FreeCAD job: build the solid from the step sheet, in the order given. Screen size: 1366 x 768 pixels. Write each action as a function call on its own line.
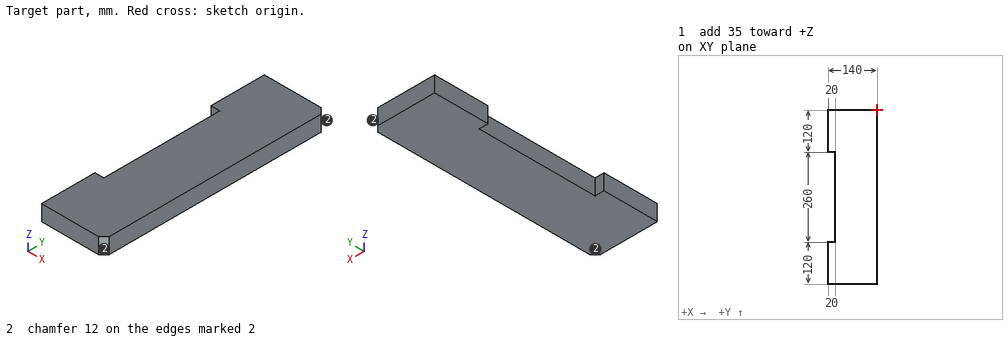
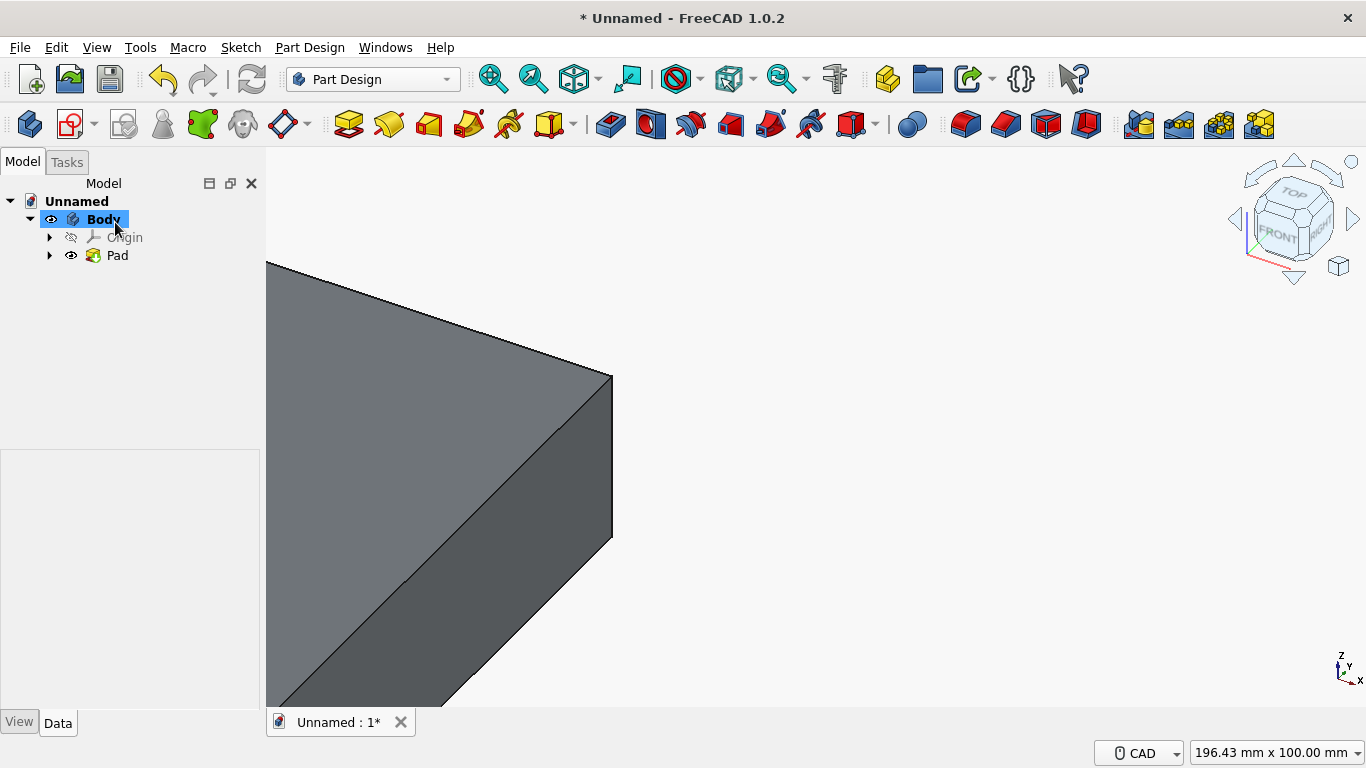
click(494, 80)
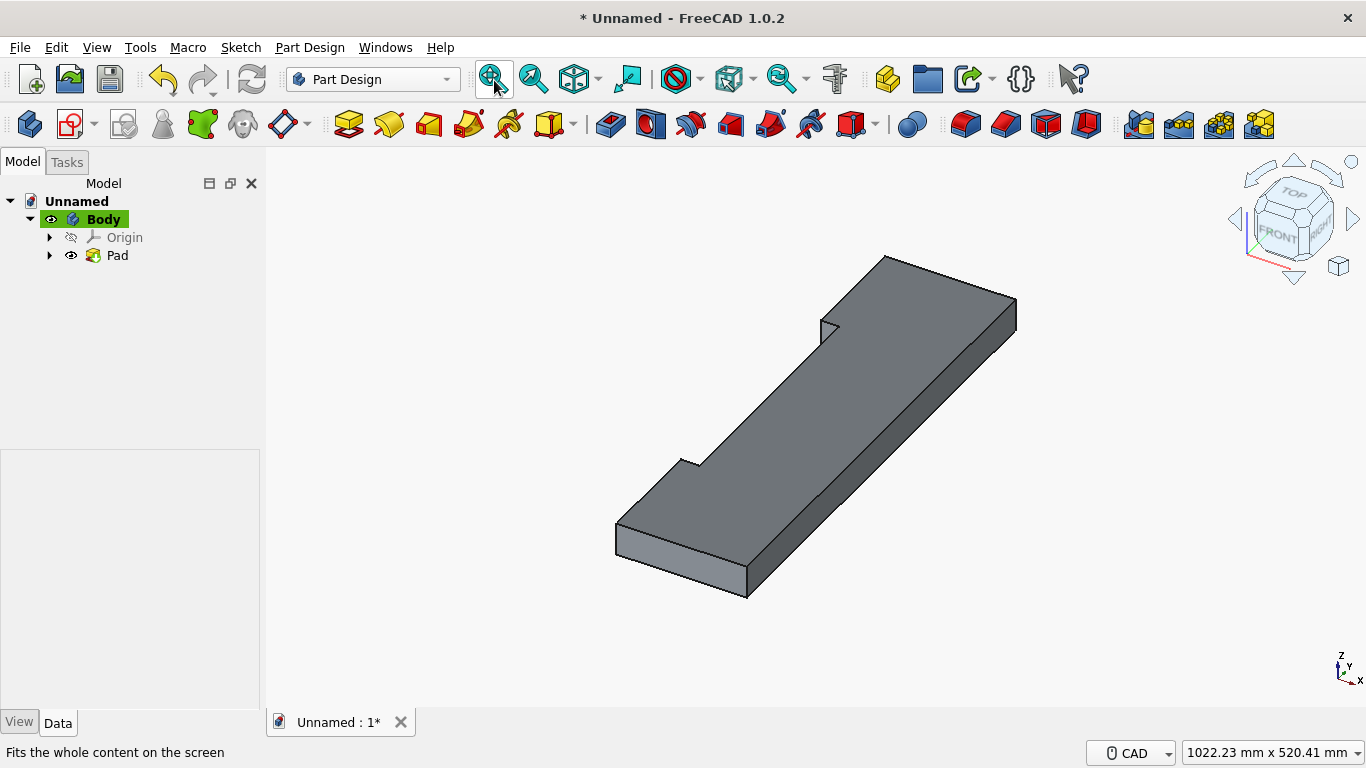
click(747, 581)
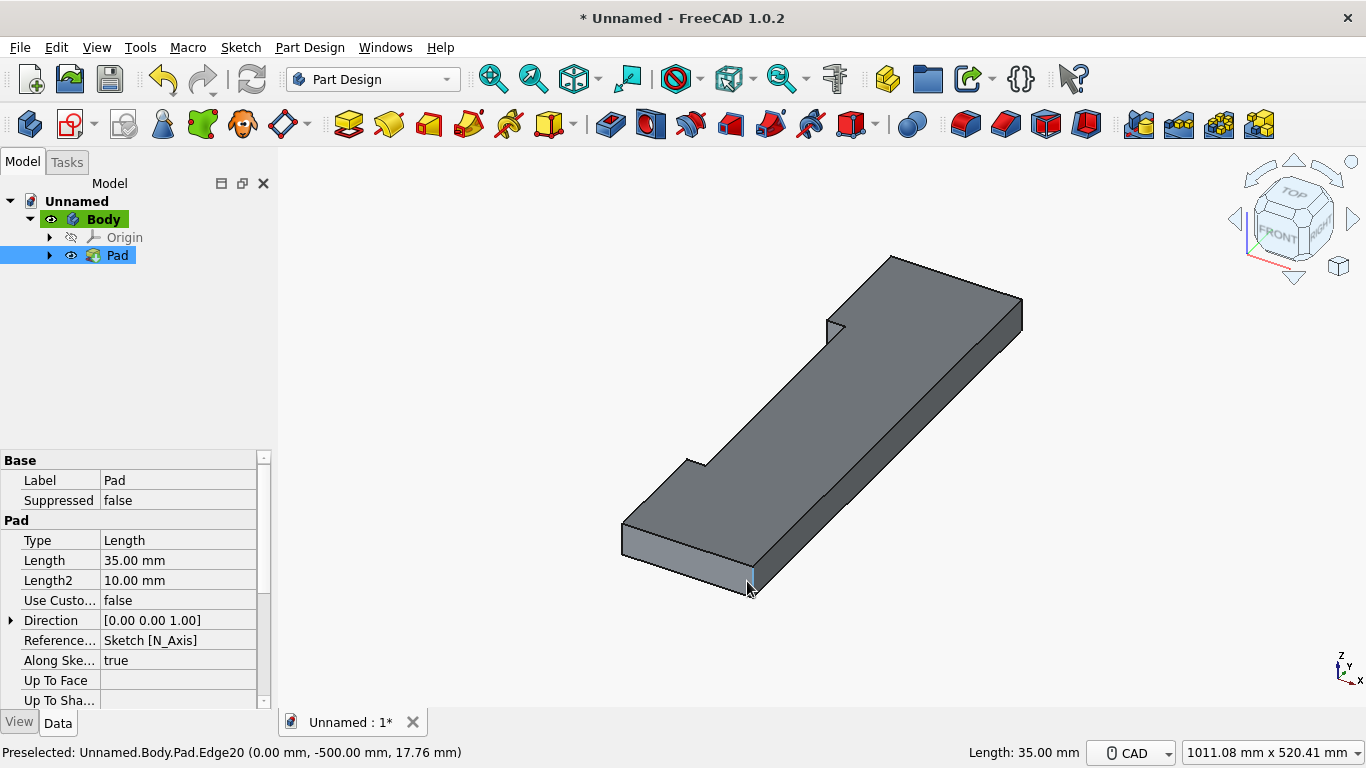
key(0)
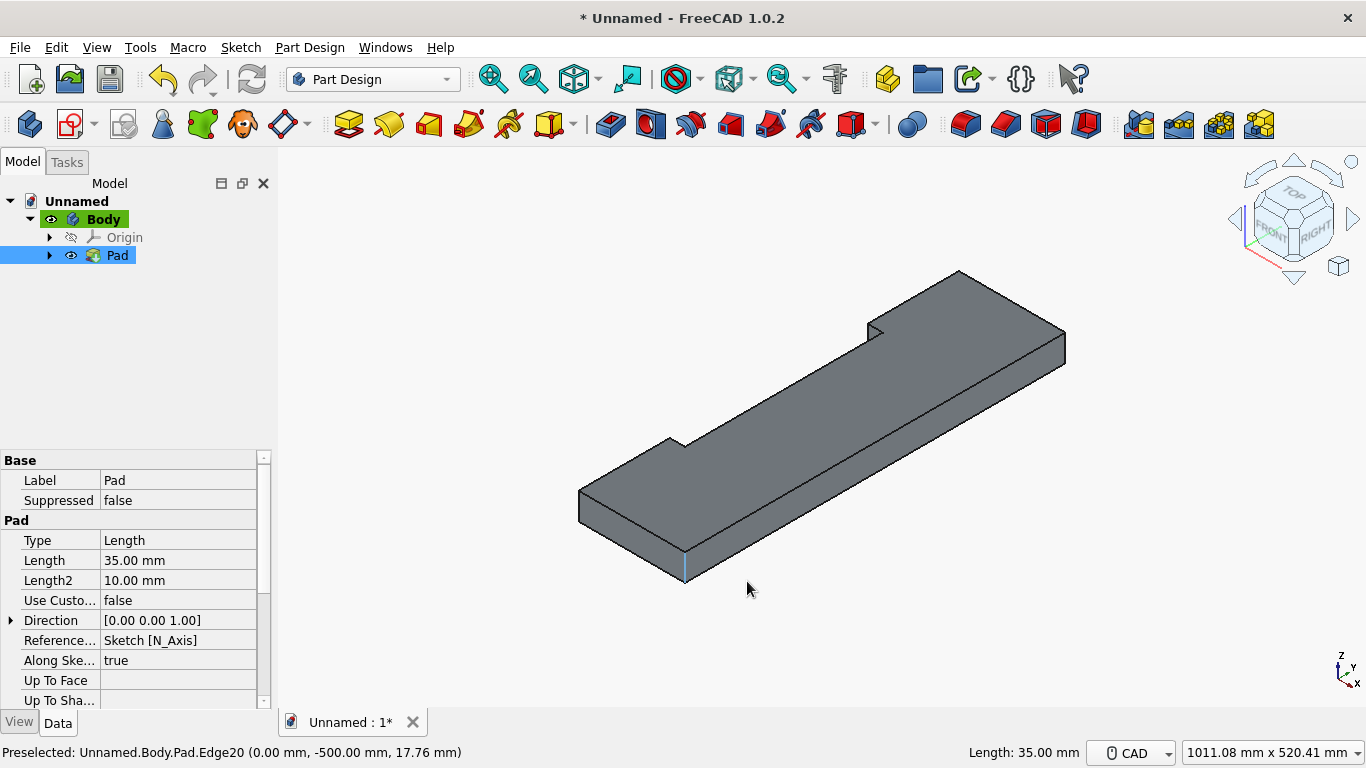
key(2)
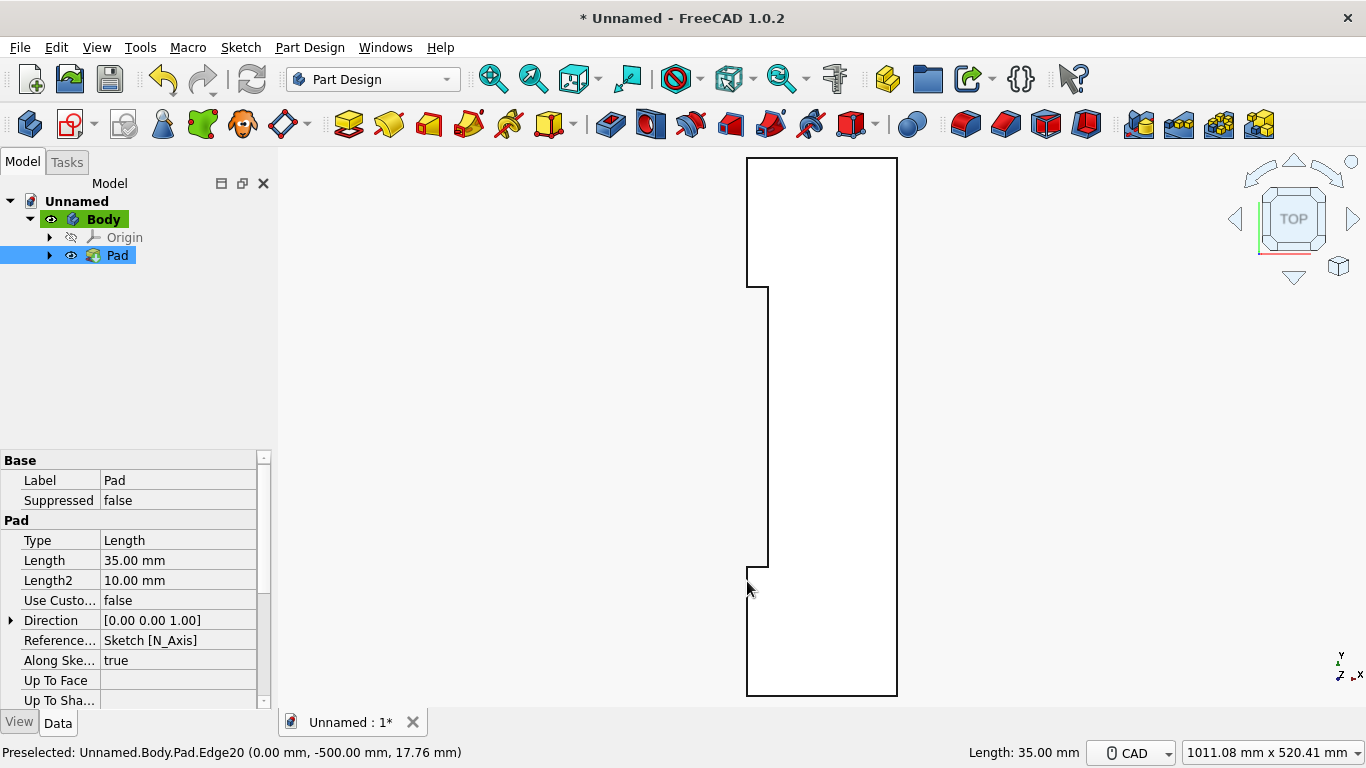
key(1)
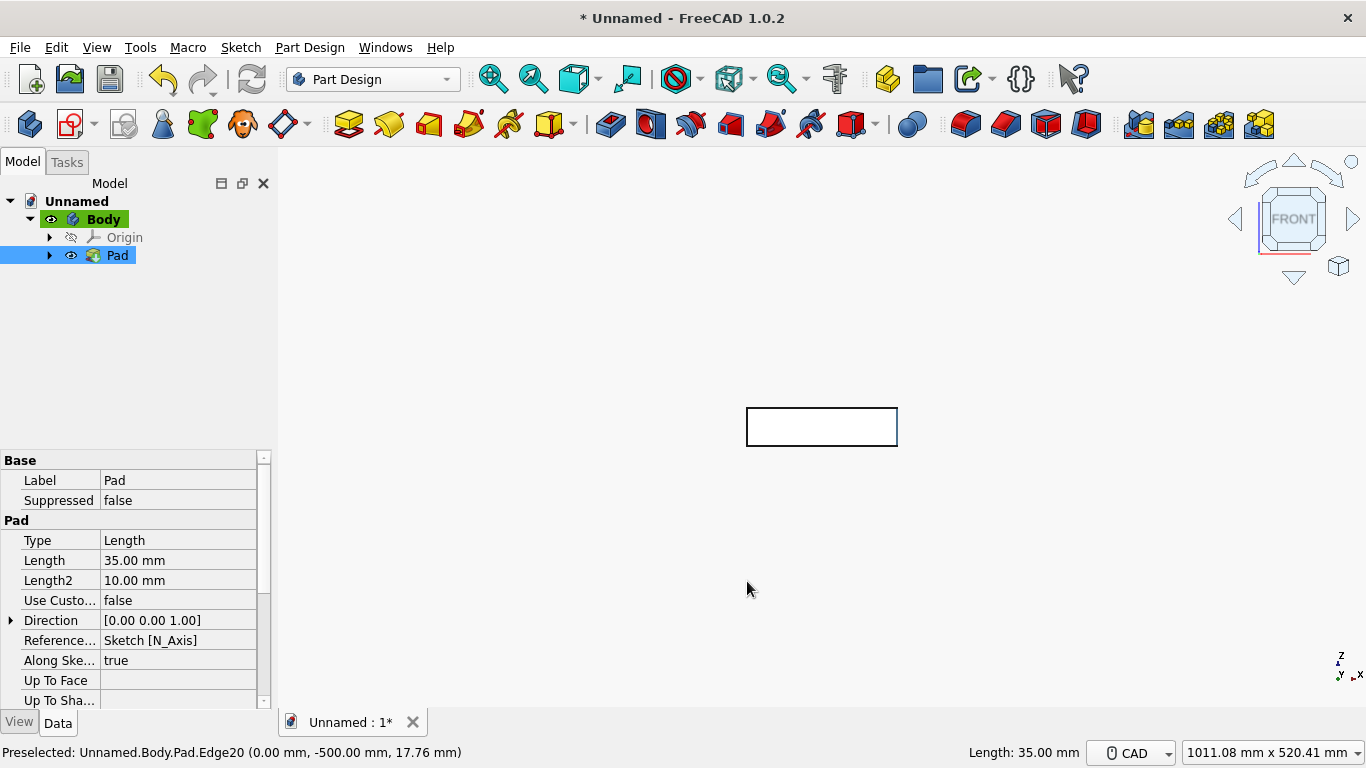
key(v)
key(f)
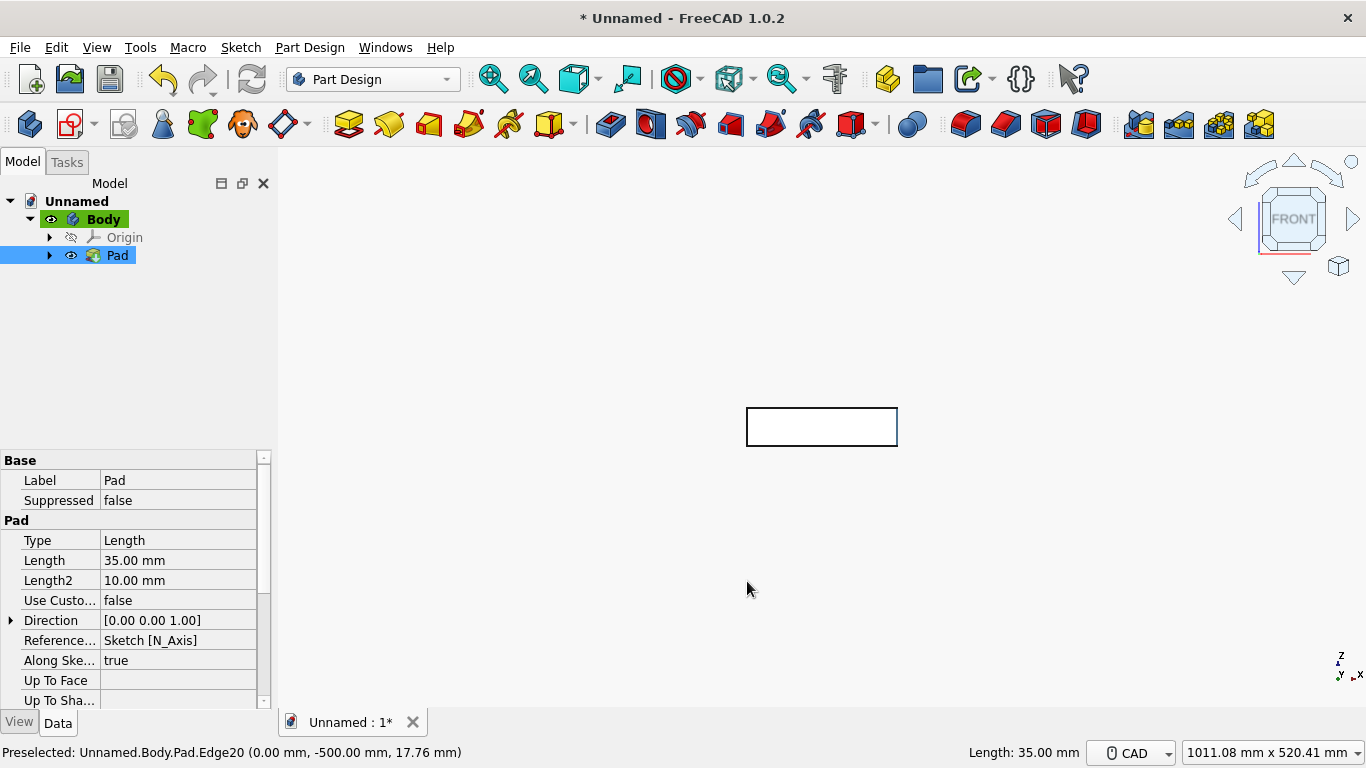
key(3)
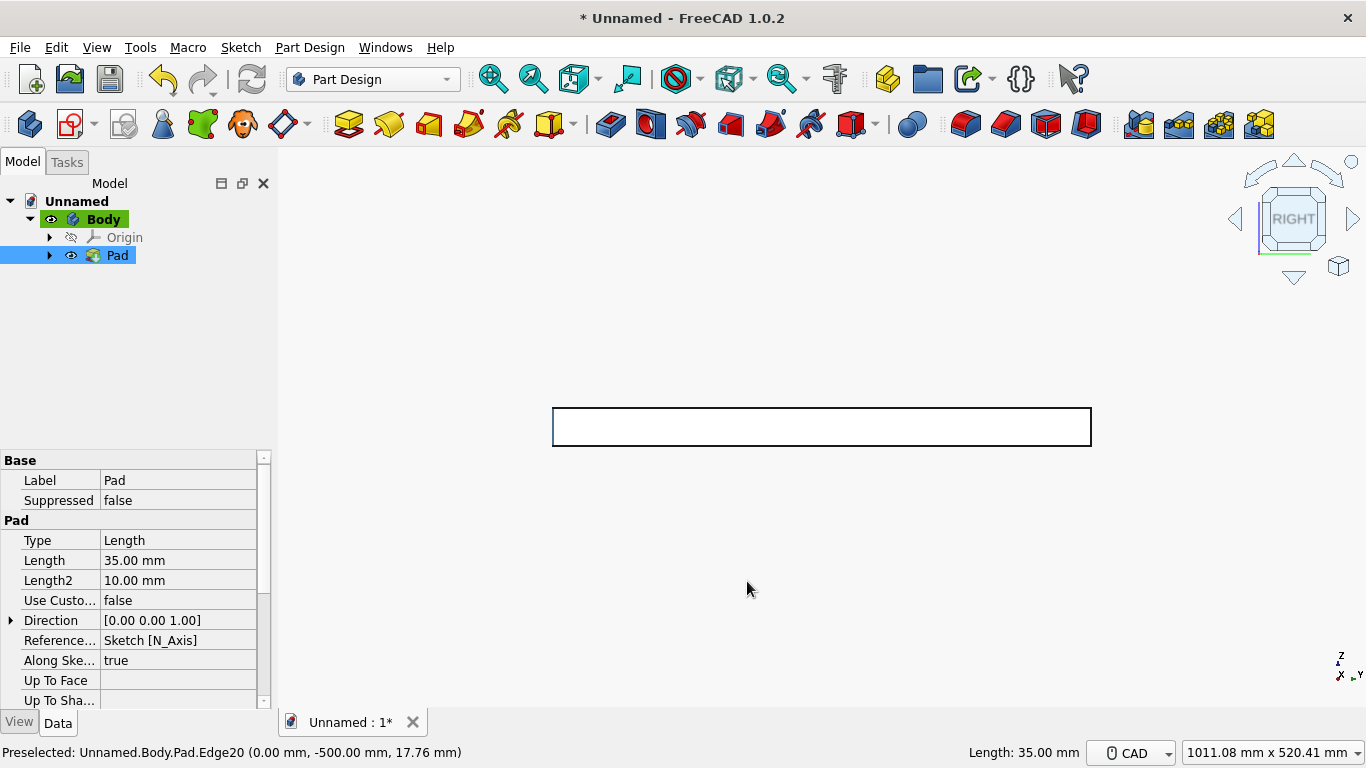
click(1091, 426, ctrl)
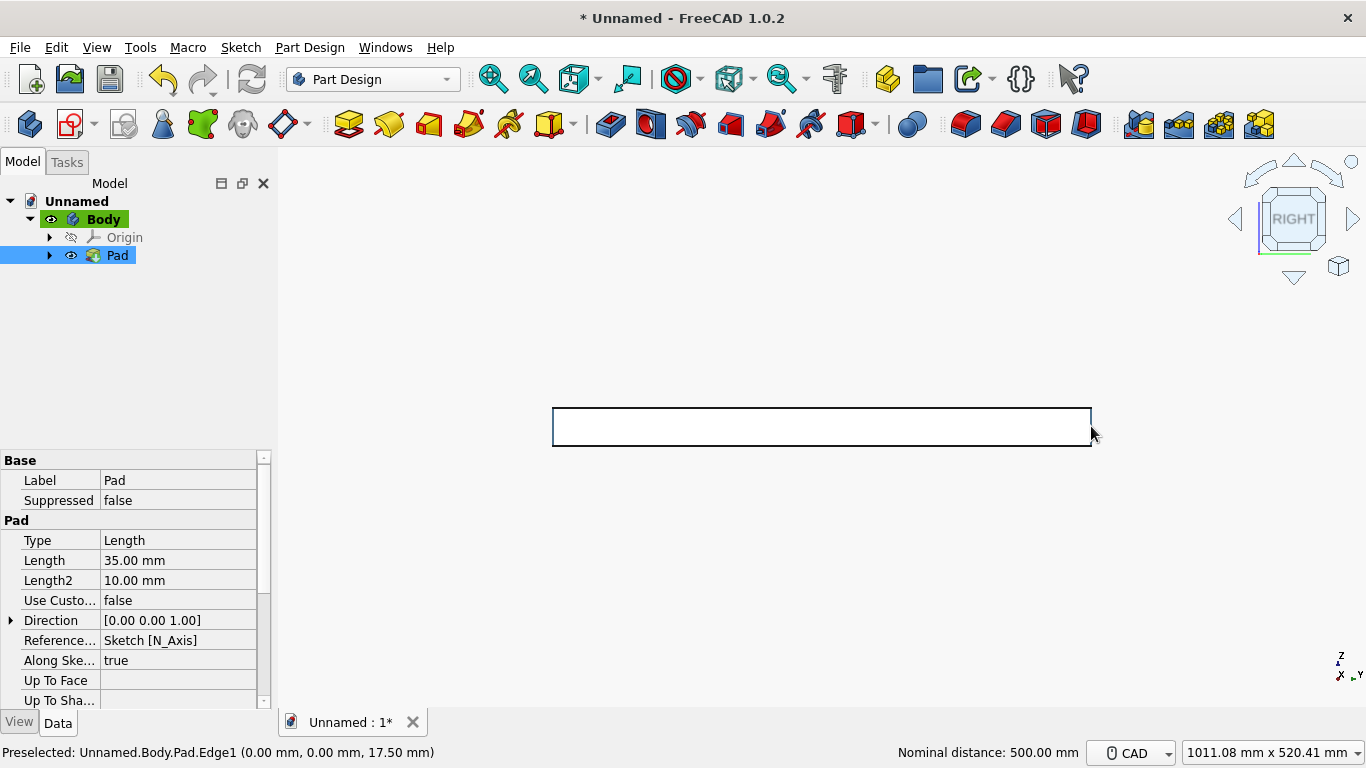
click(1006, 124)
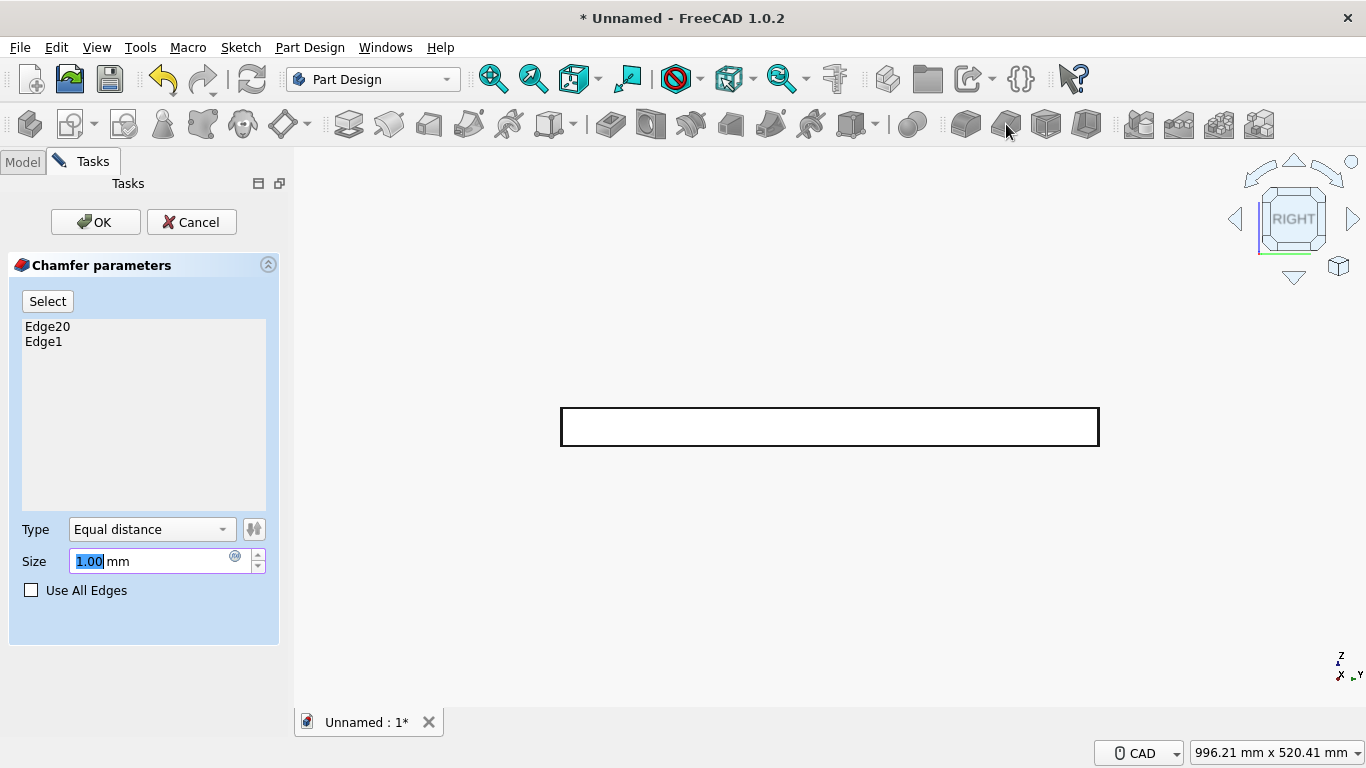
text(12)
key(Tab)